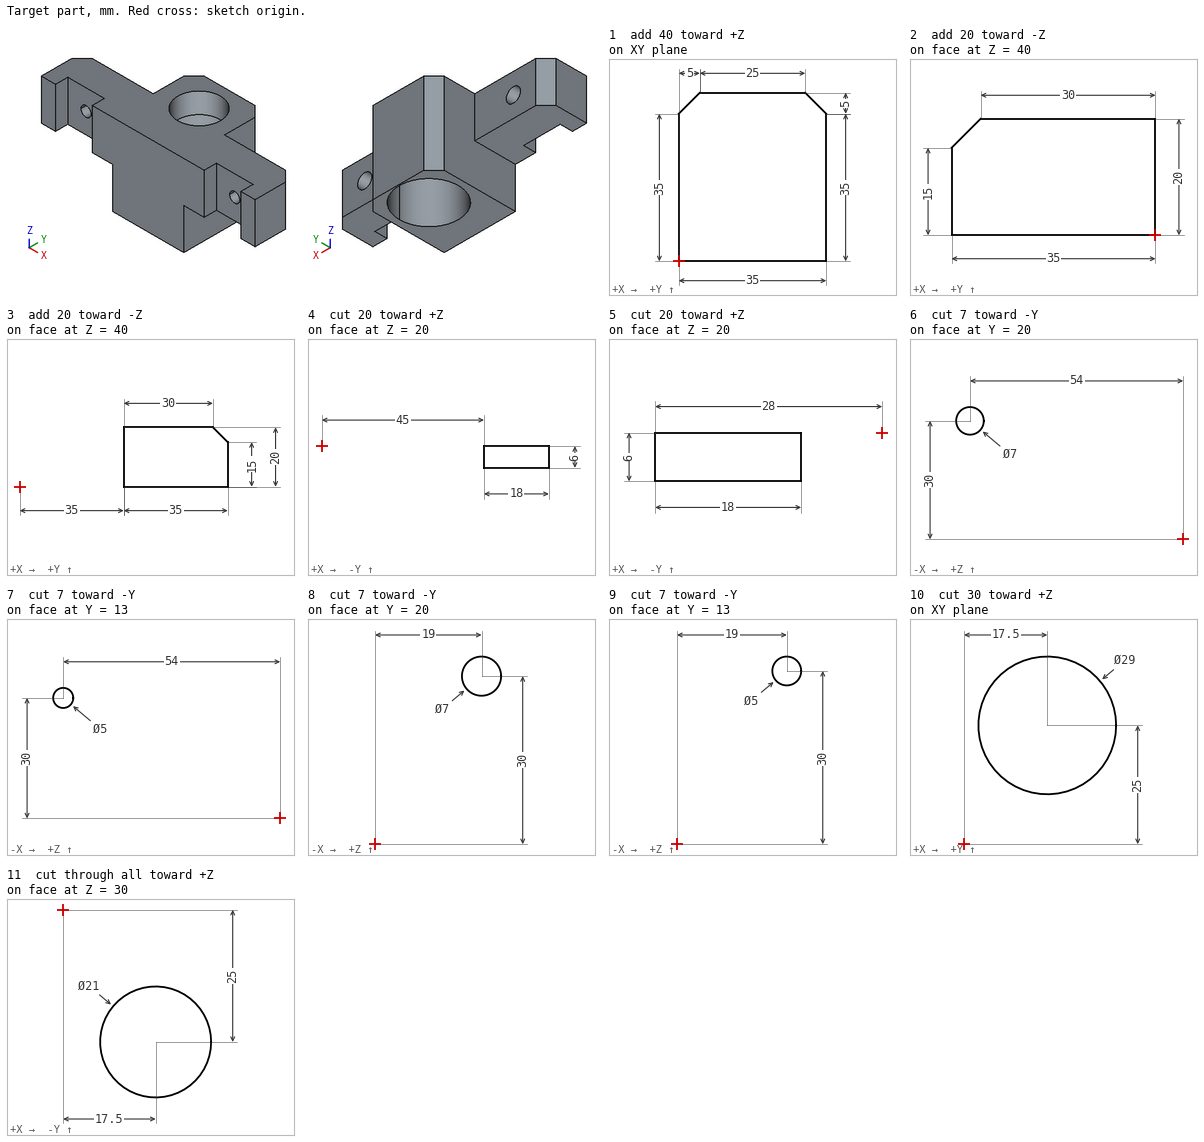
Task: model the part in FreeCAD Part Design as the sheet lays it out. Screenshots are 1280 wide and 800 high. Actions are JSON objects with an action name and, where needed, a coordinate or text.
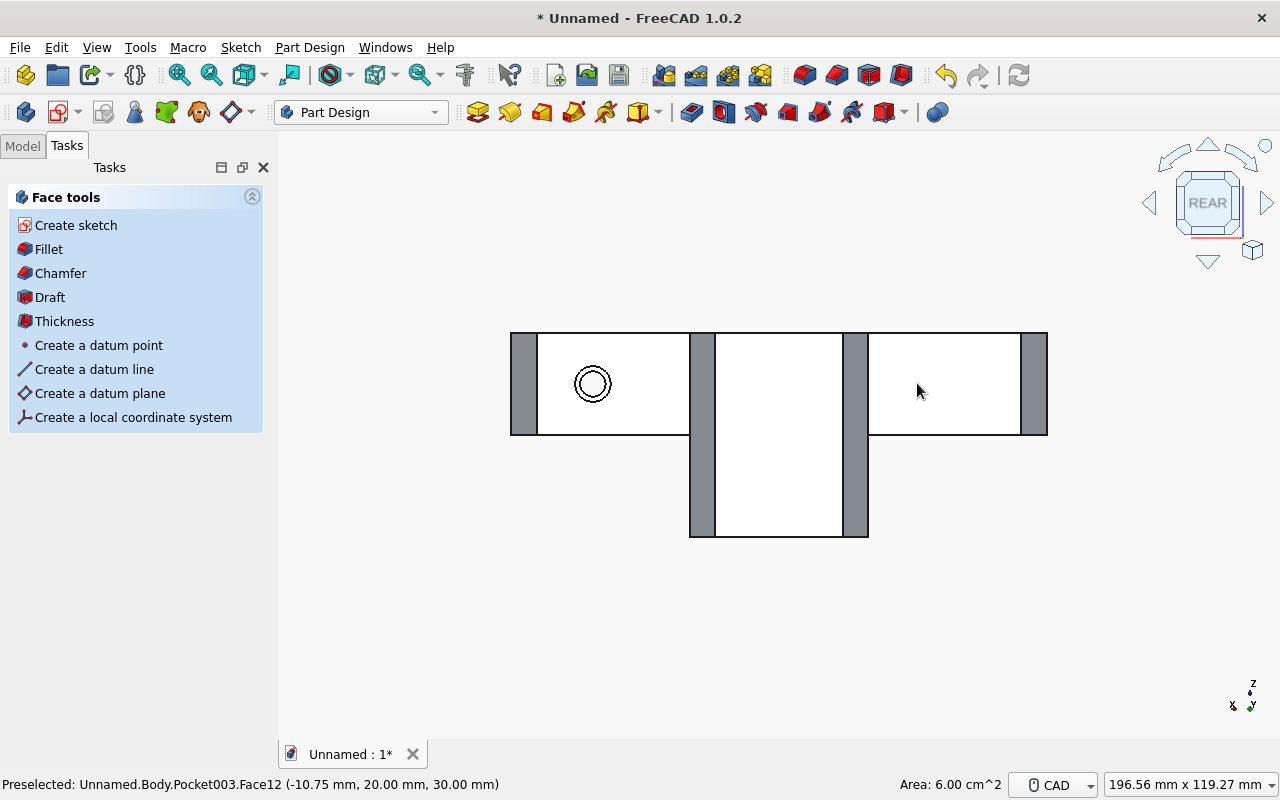
{"action": "left_click", "coordinate": [58, 112]}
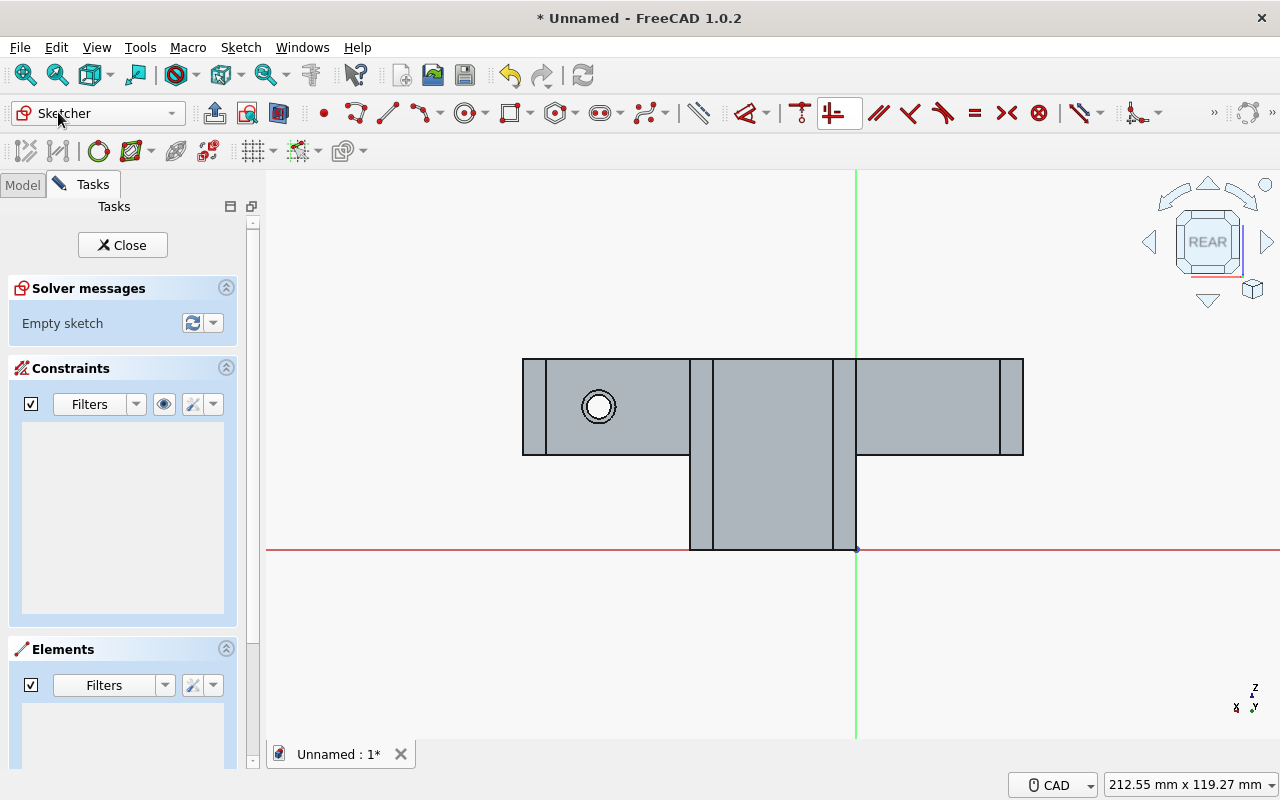
{"action": "left_click", "coordinate": [280, 114]}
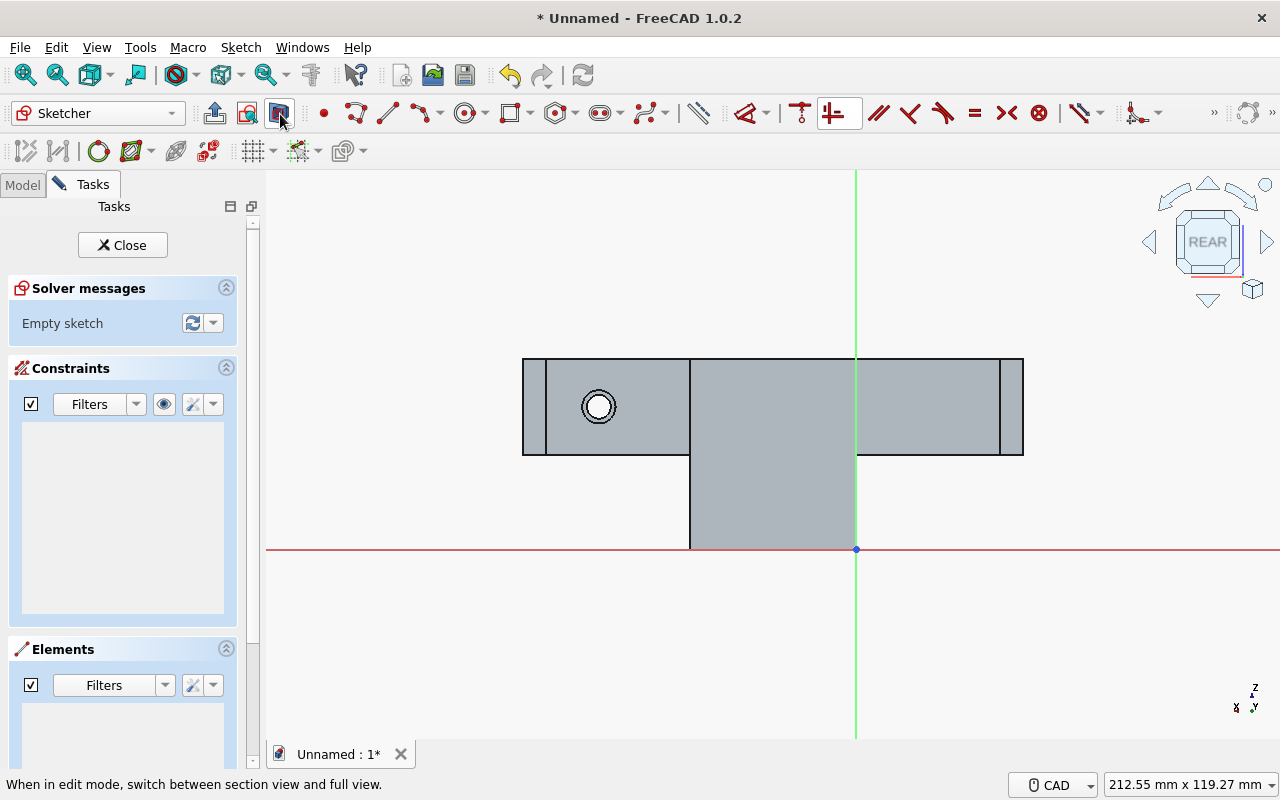
{"action": "scroll", "coordinate": [971, 402], "scroll_direction": "up", "scroll_amount": 12}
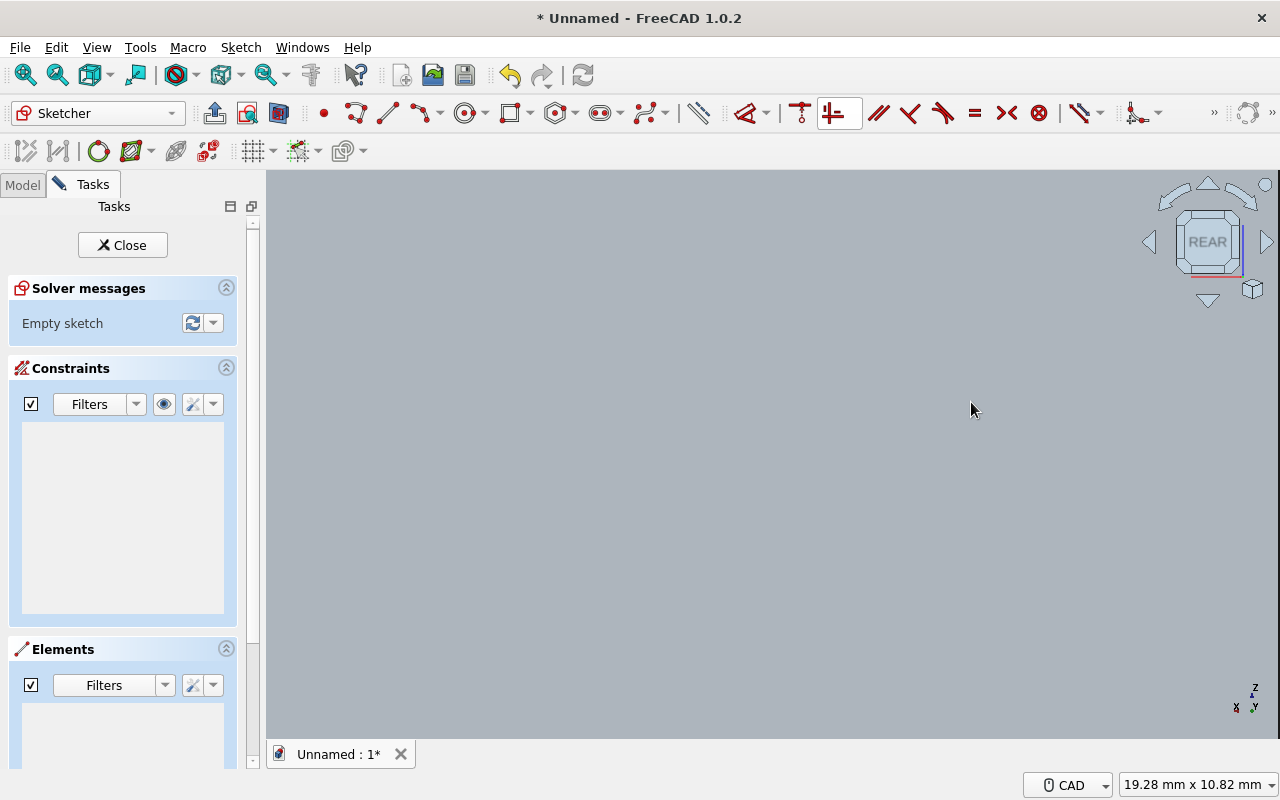
{"action": "left_click", "coordinate": [466, 114]}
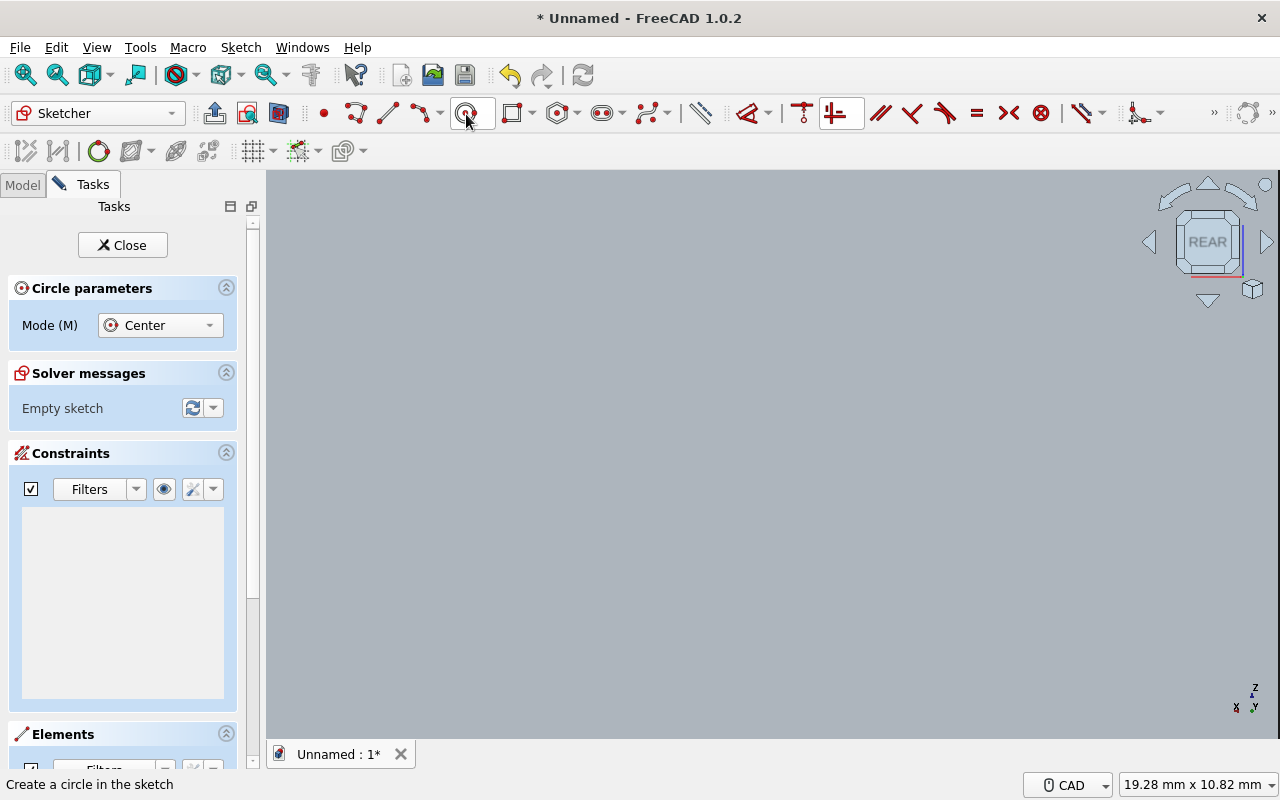
{"action": "left_click", "coordinate": [701, 451]}
{"action": "left_click", "coordinate": [831, 321]}
{"action": "key", "text": "Escape"}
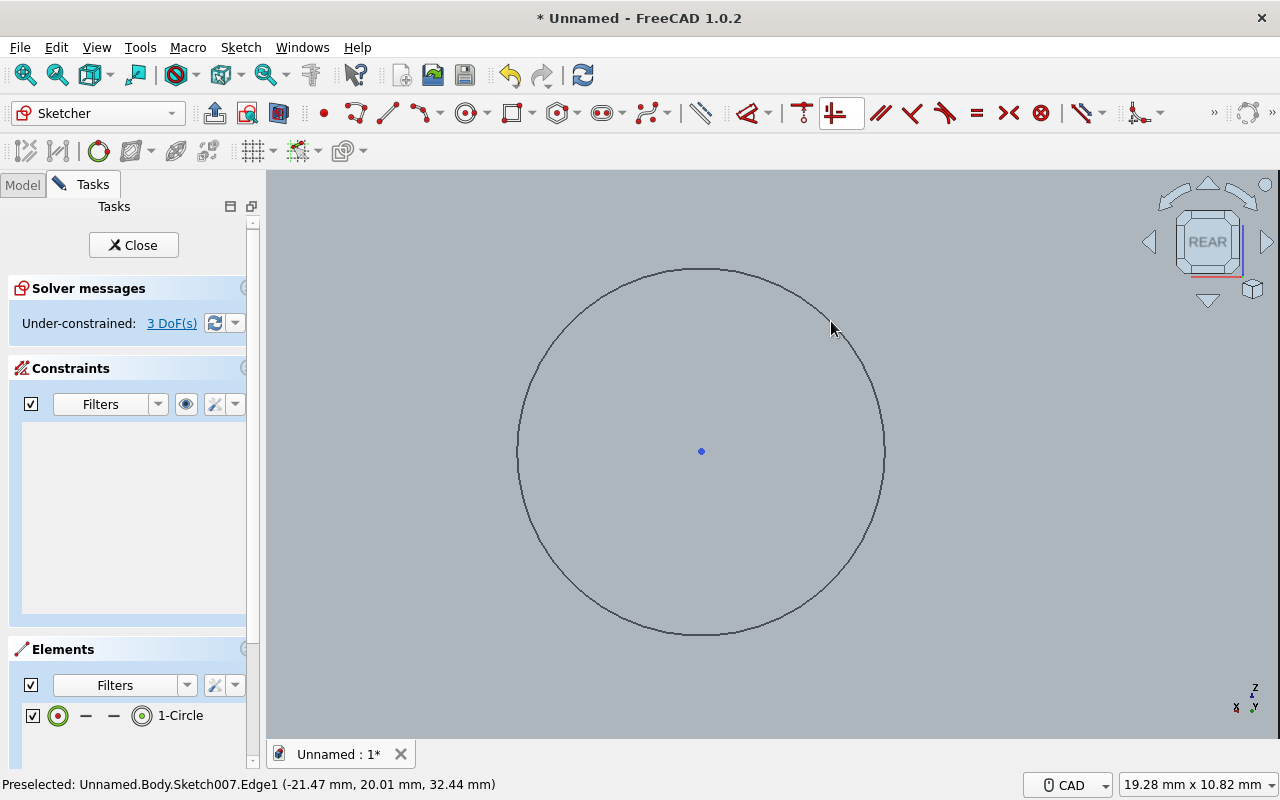
{"action": "left_click", "coordinate": [748, 114]}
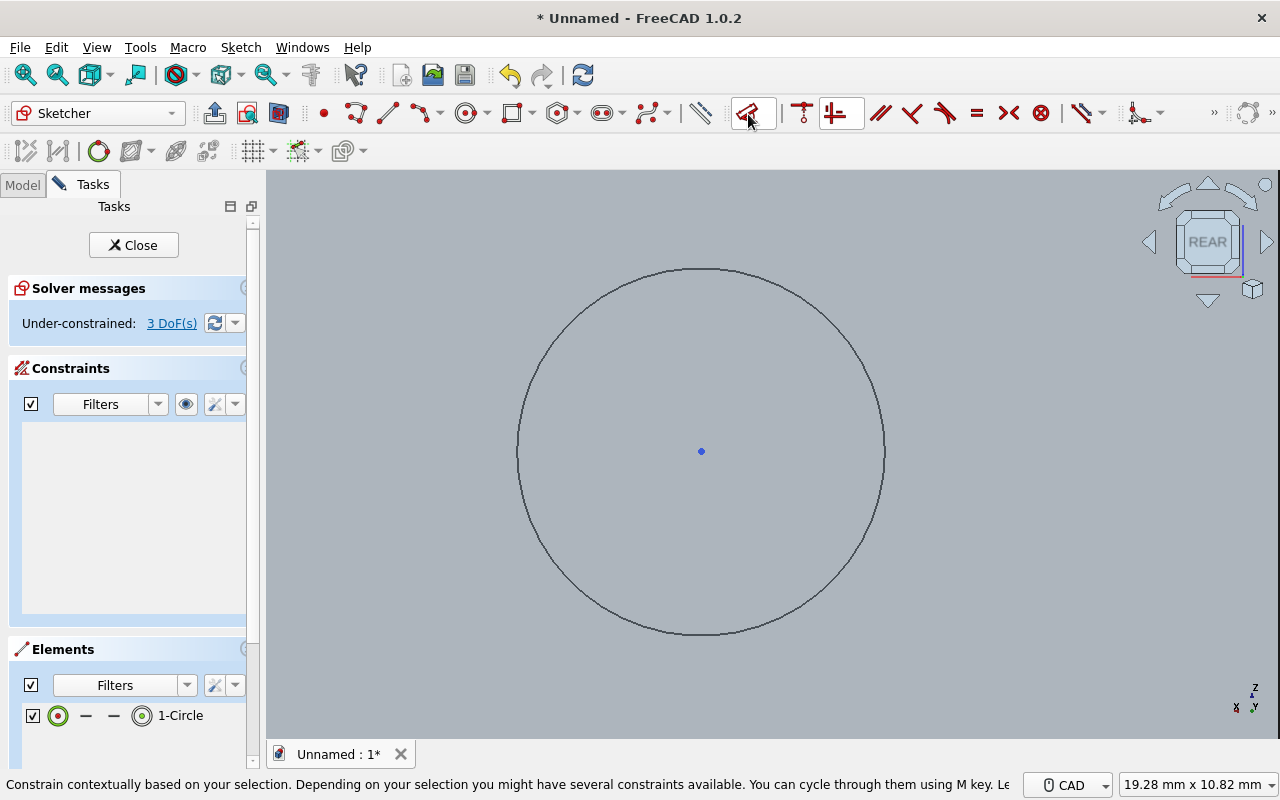
{"action": "left_click", "coordinate": [831, 322]}
{"action": "left_click", "coordinate": [854, 299]}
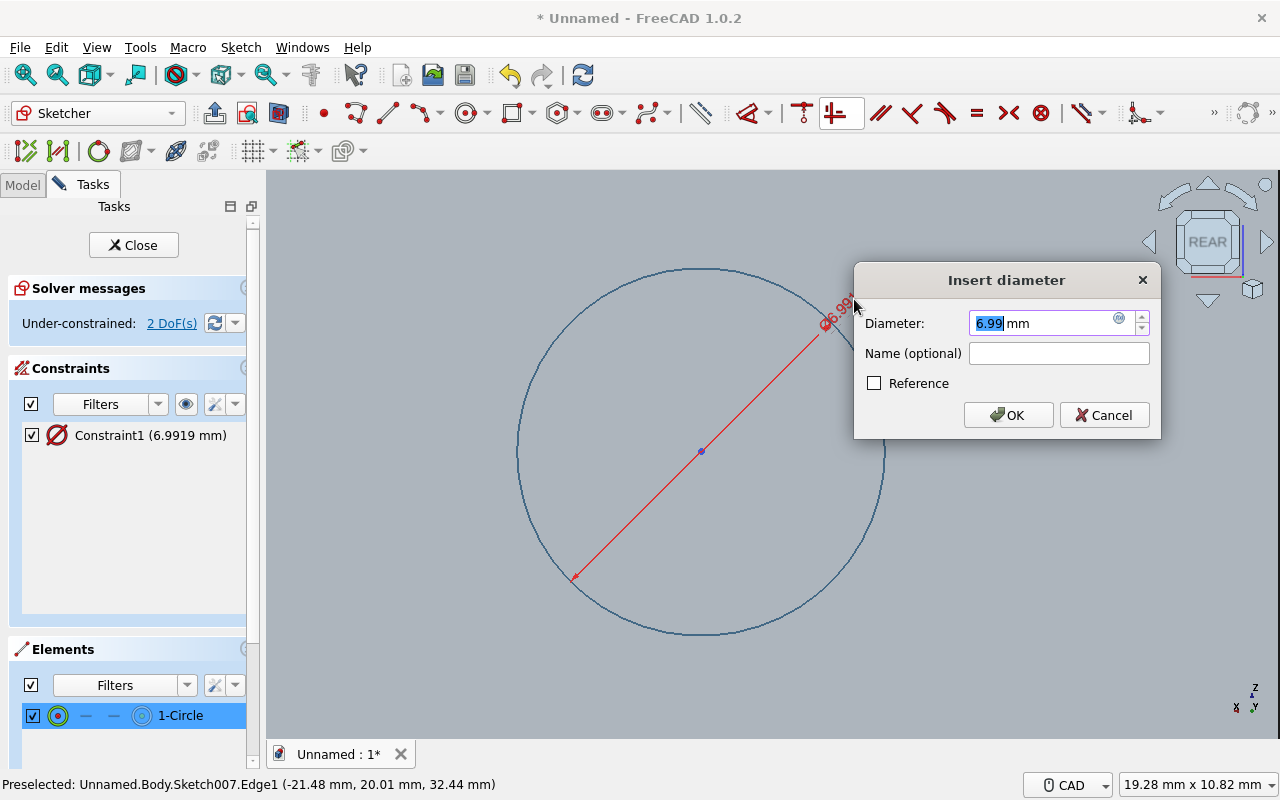
{"action": "type", "text": "7"}
{"action": "key", "text": "Return"}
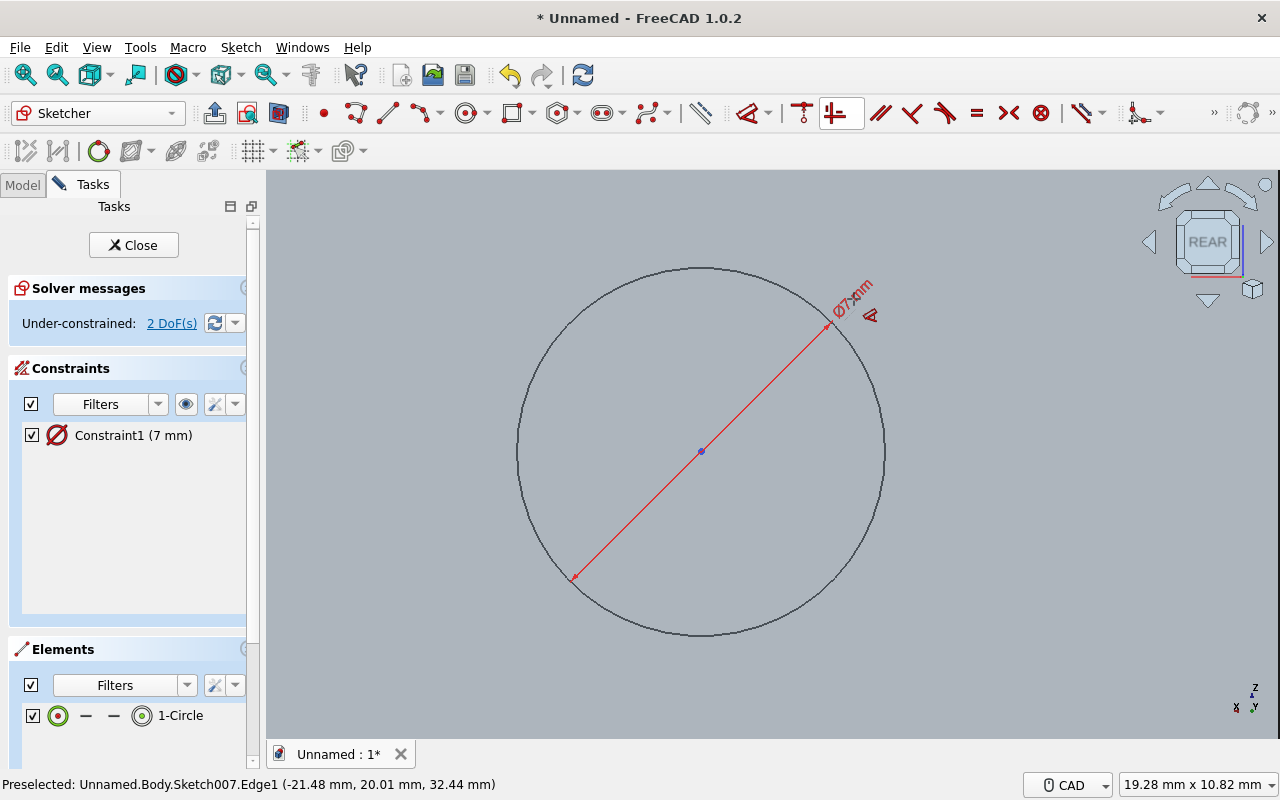
{"action": "left_click", "coordinate": [701, 452]}
{"action": "left_click", "coordinate": [498, 418]}